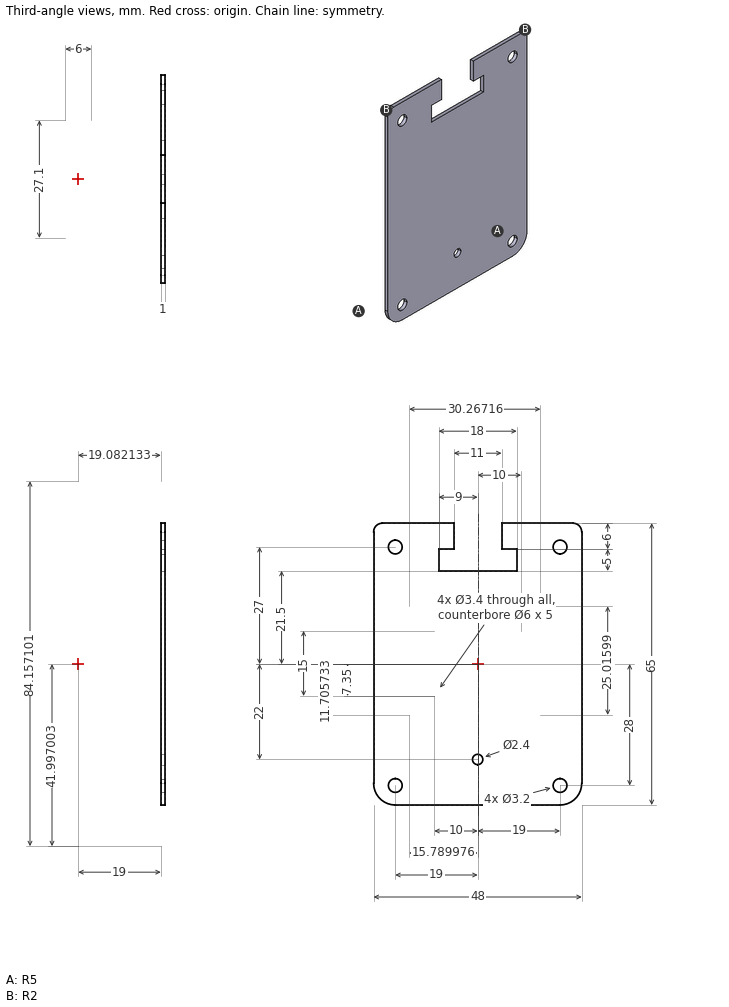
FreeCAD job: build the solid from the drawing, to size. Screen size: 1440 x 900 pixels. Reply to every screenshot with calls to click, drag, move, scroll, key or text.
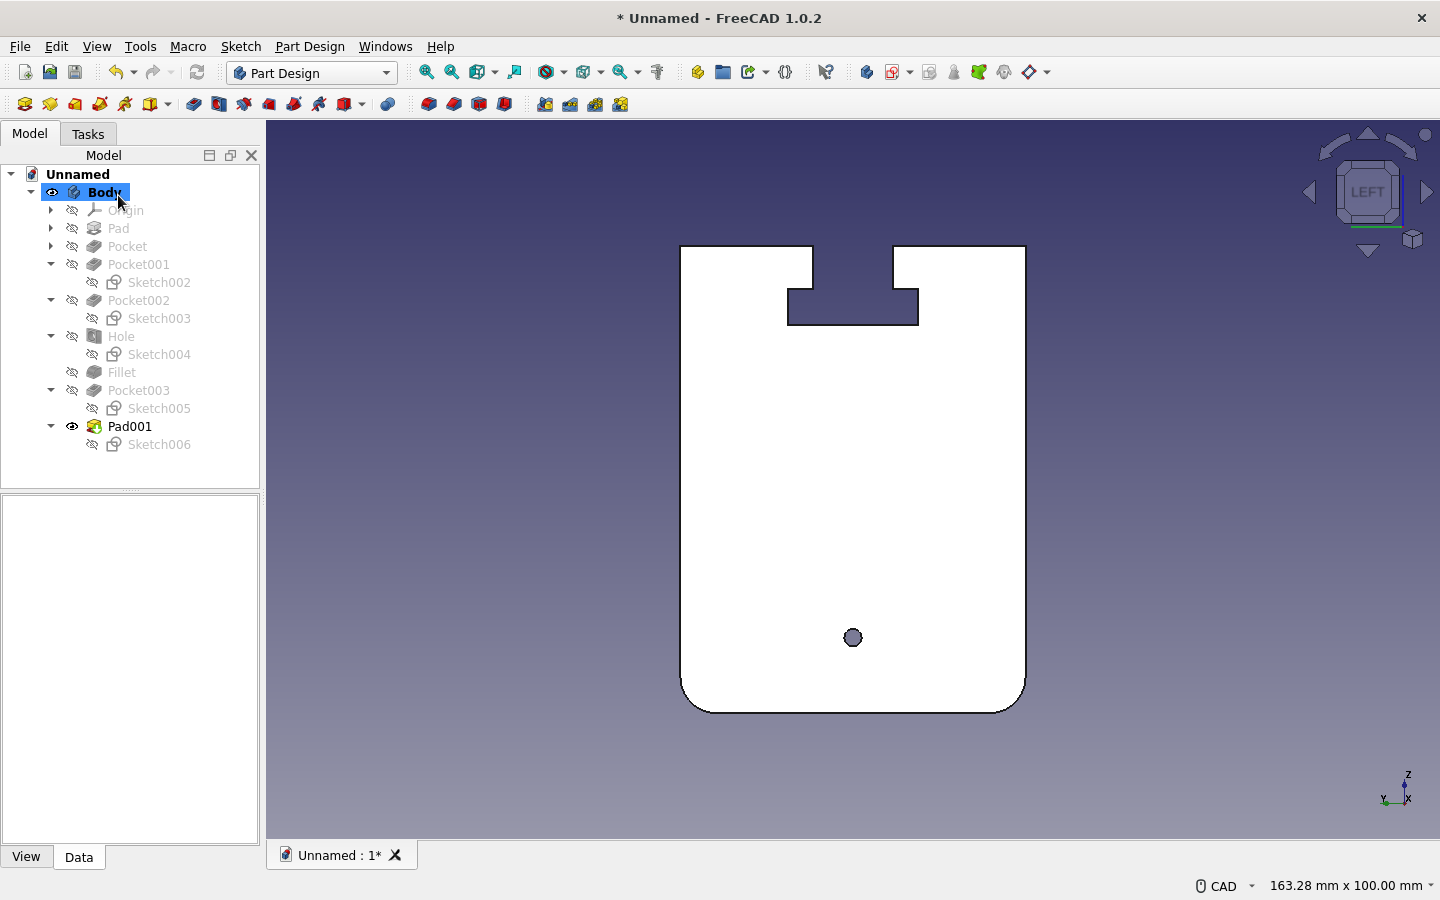
click(853, 479)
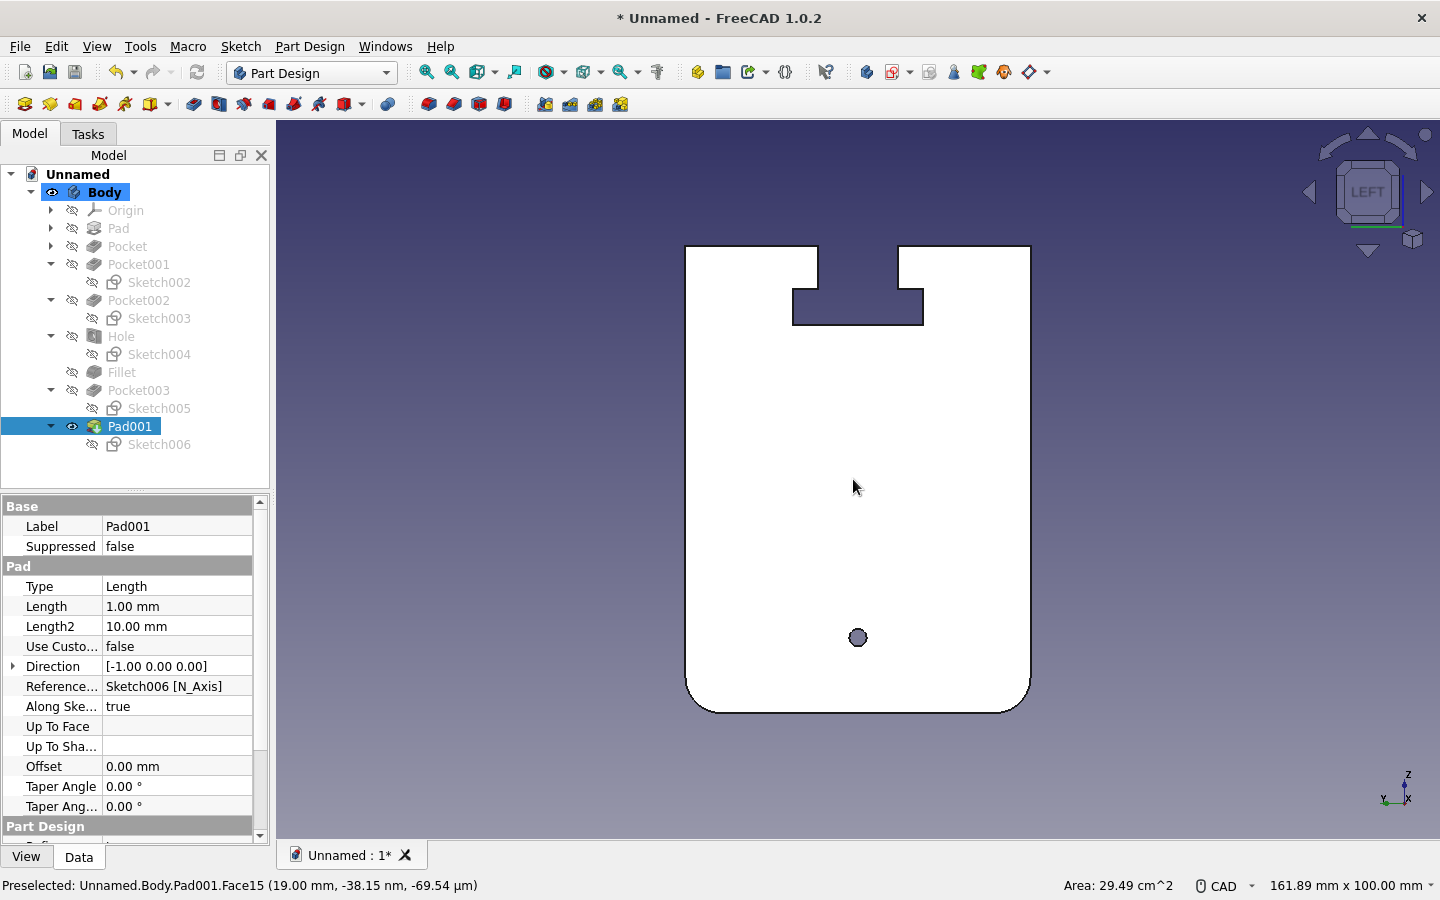
click(892, 72)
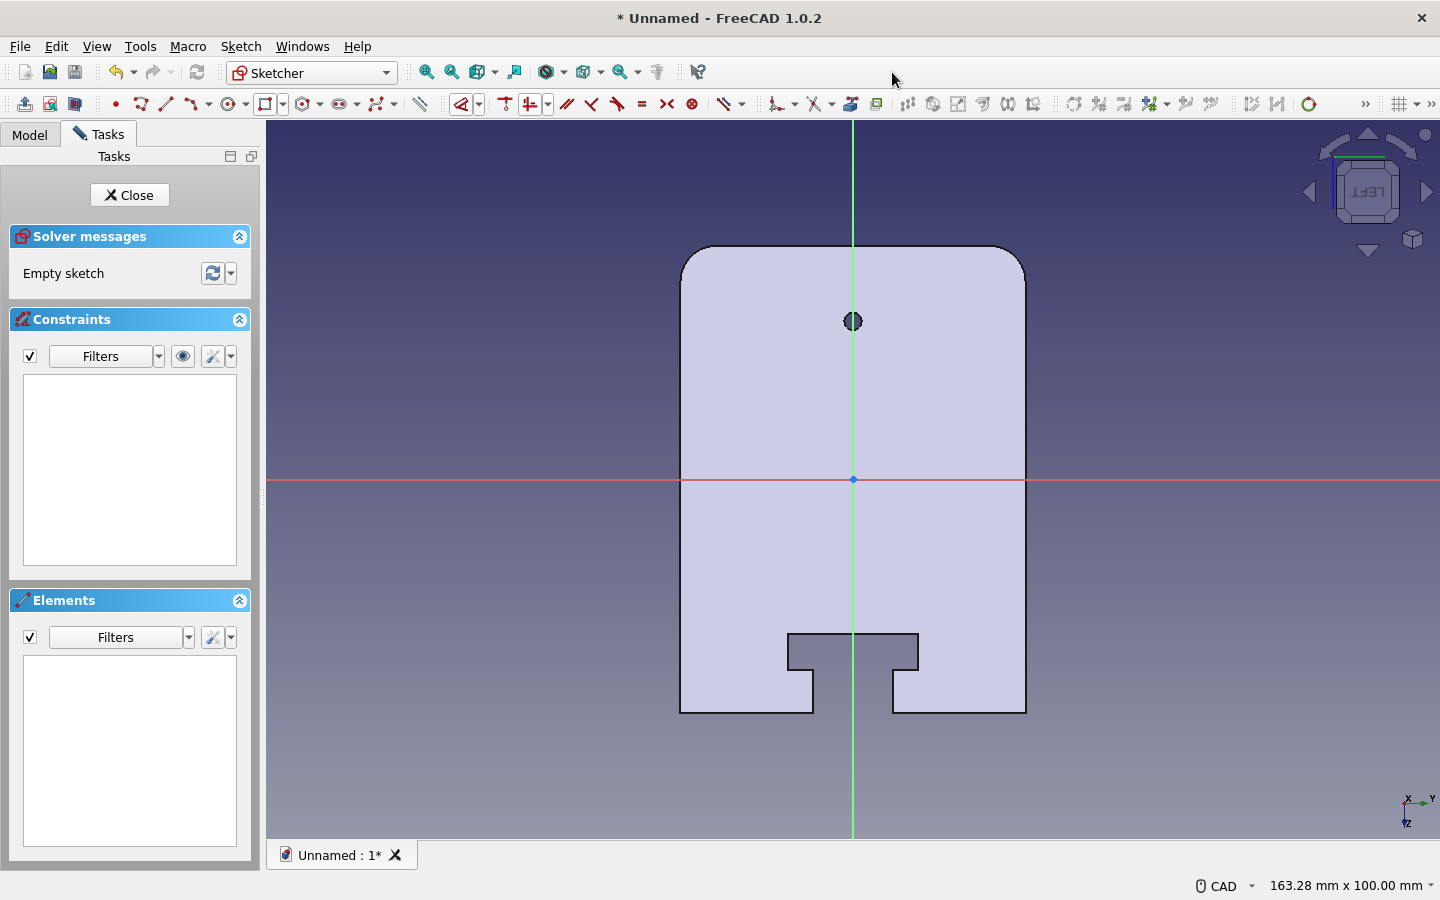
key(g)
key(c)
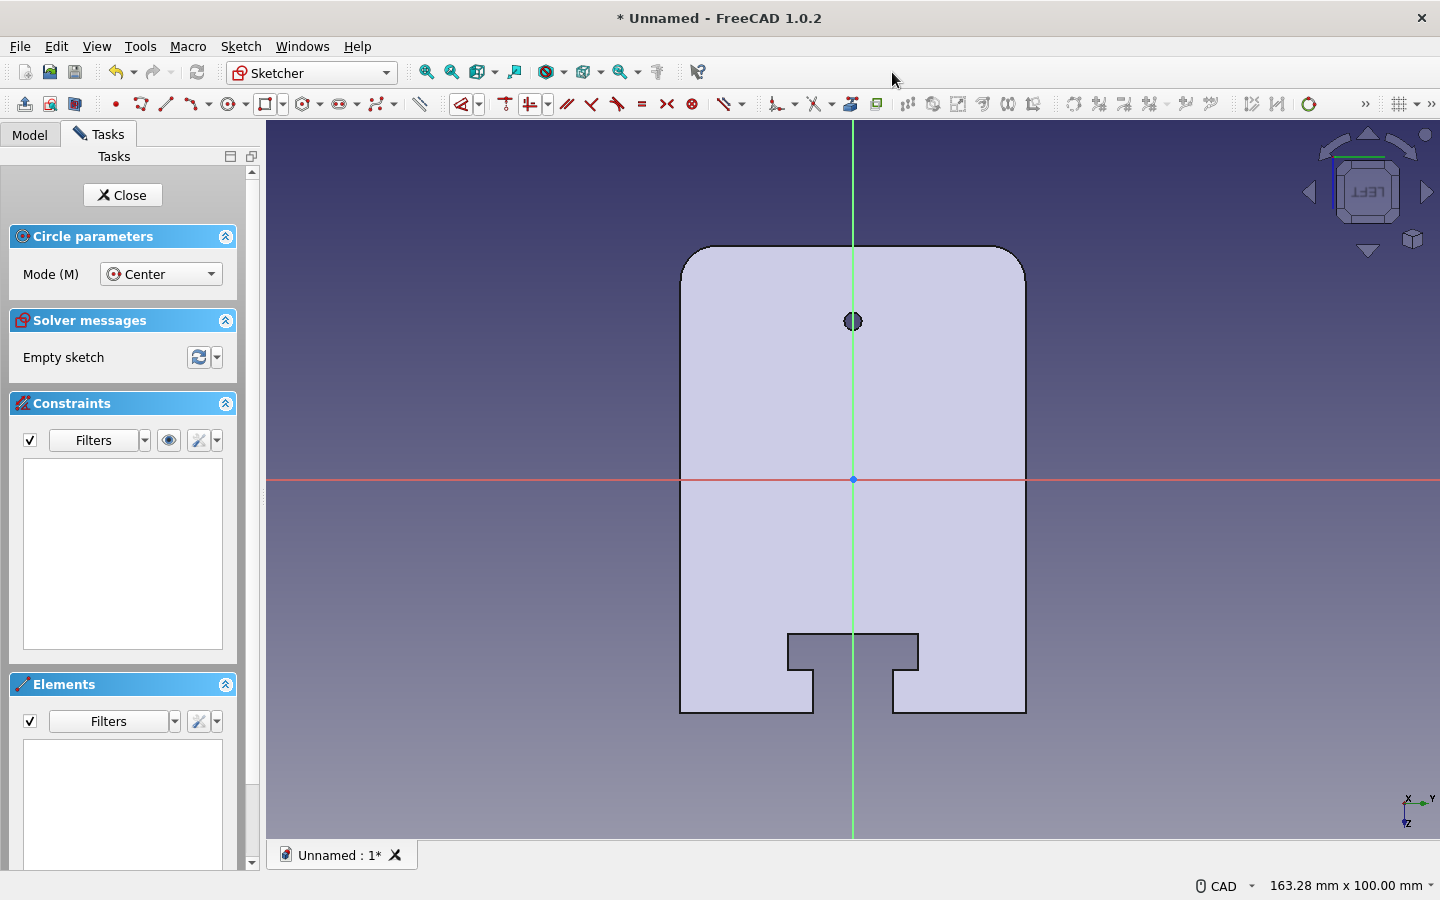
scroll(990, 278, up, 4)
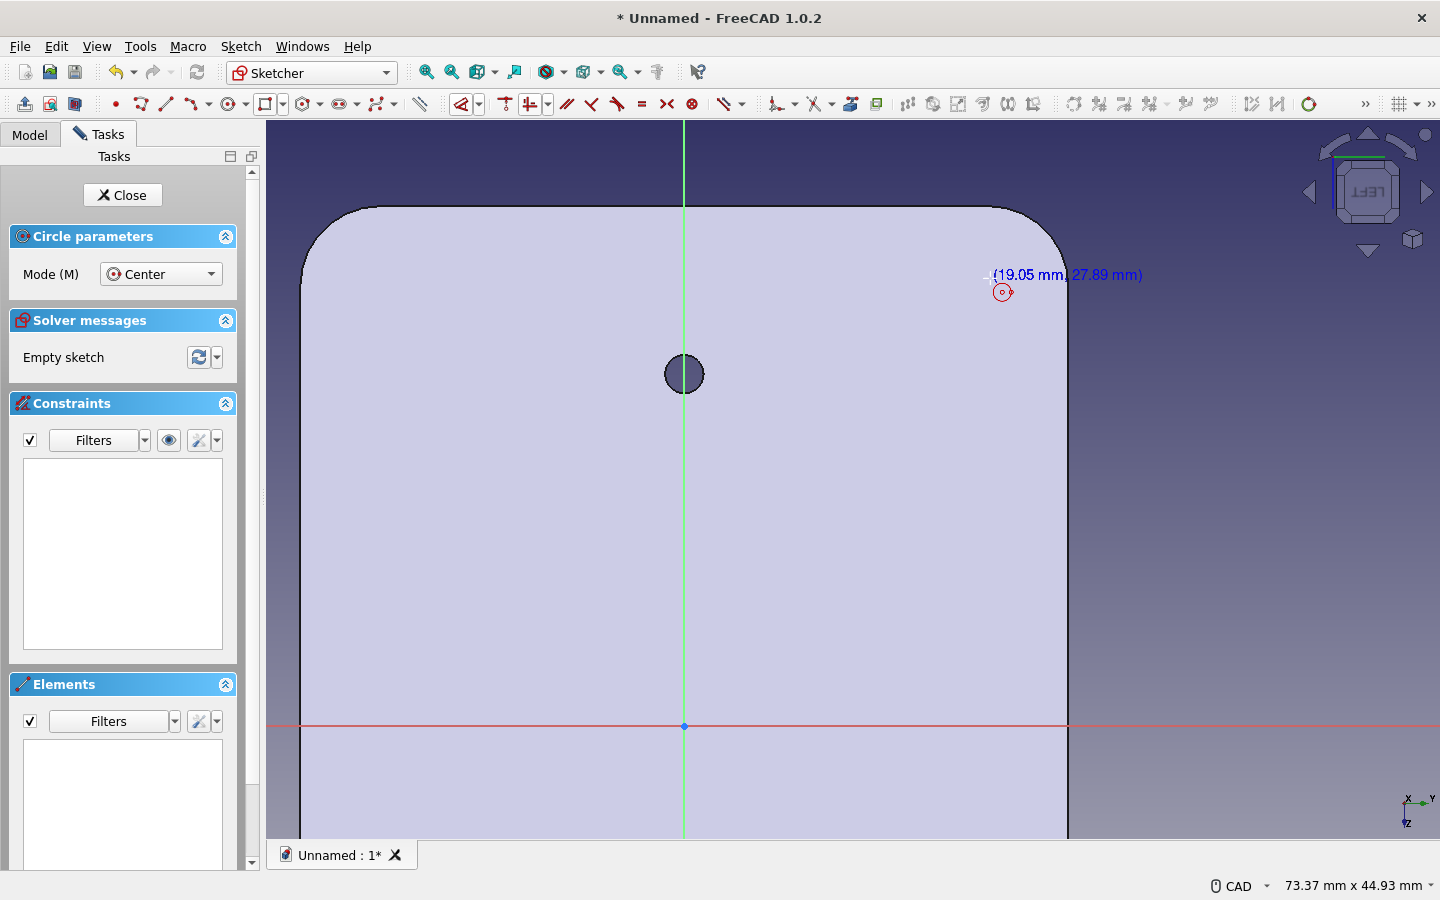
click(988, 278)
move(1006, 260)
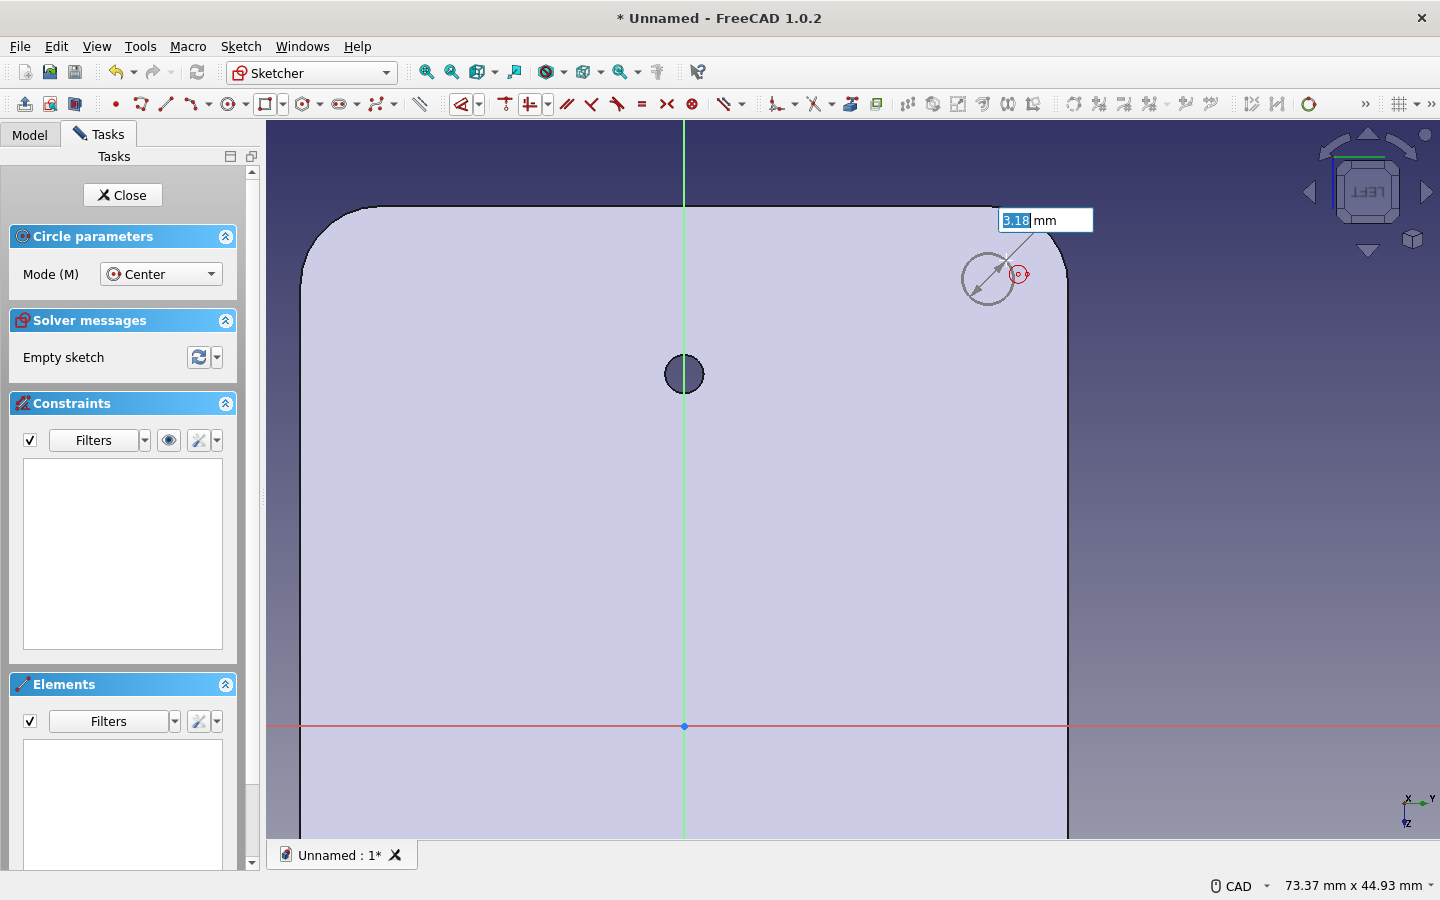
text(3.2)
key(Return)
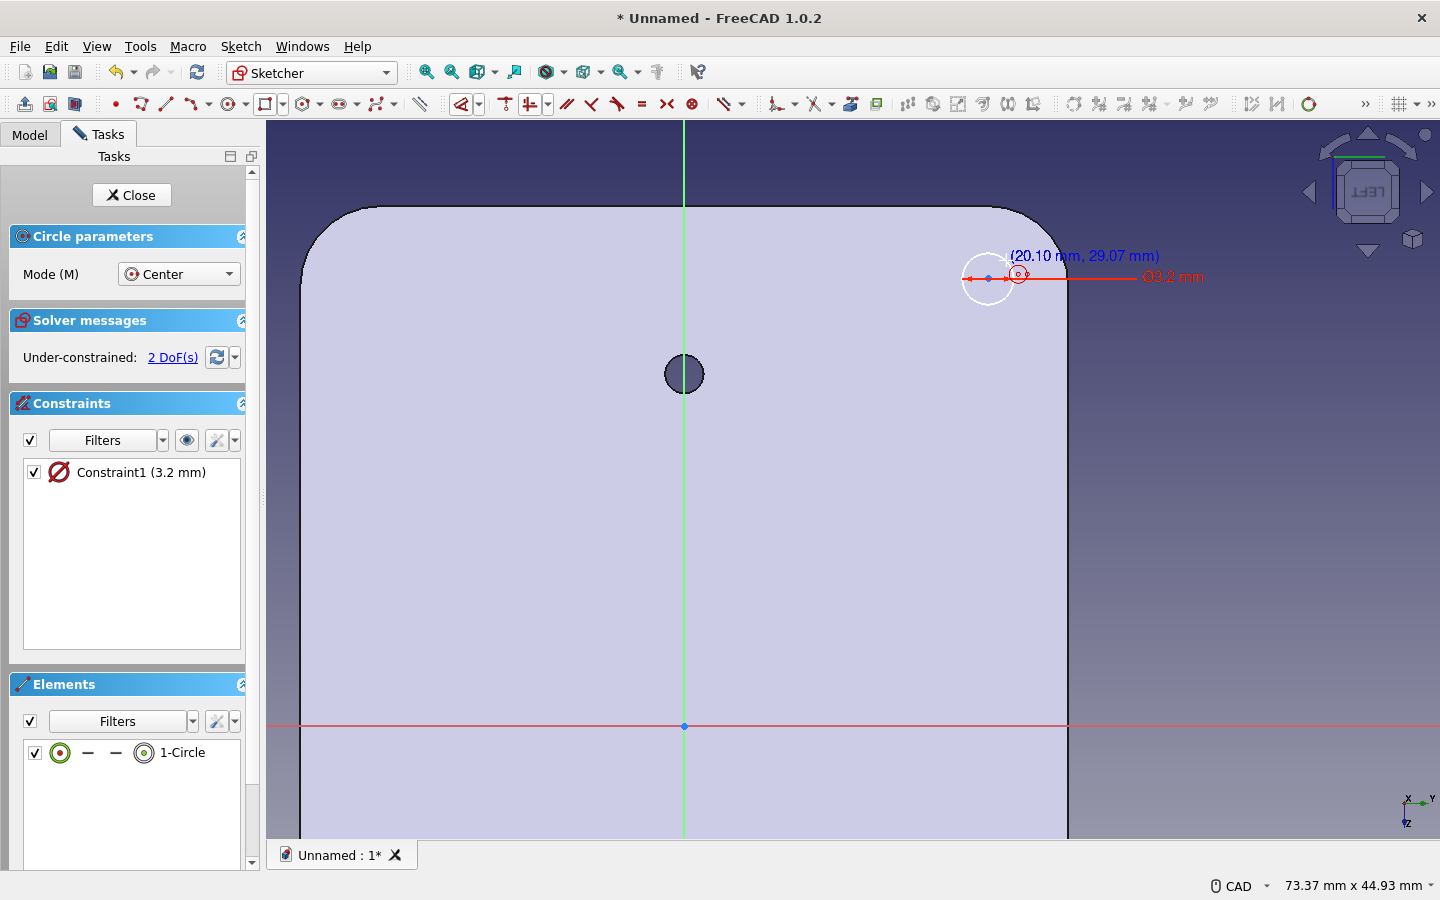
click(380, 278)
move(398, 260)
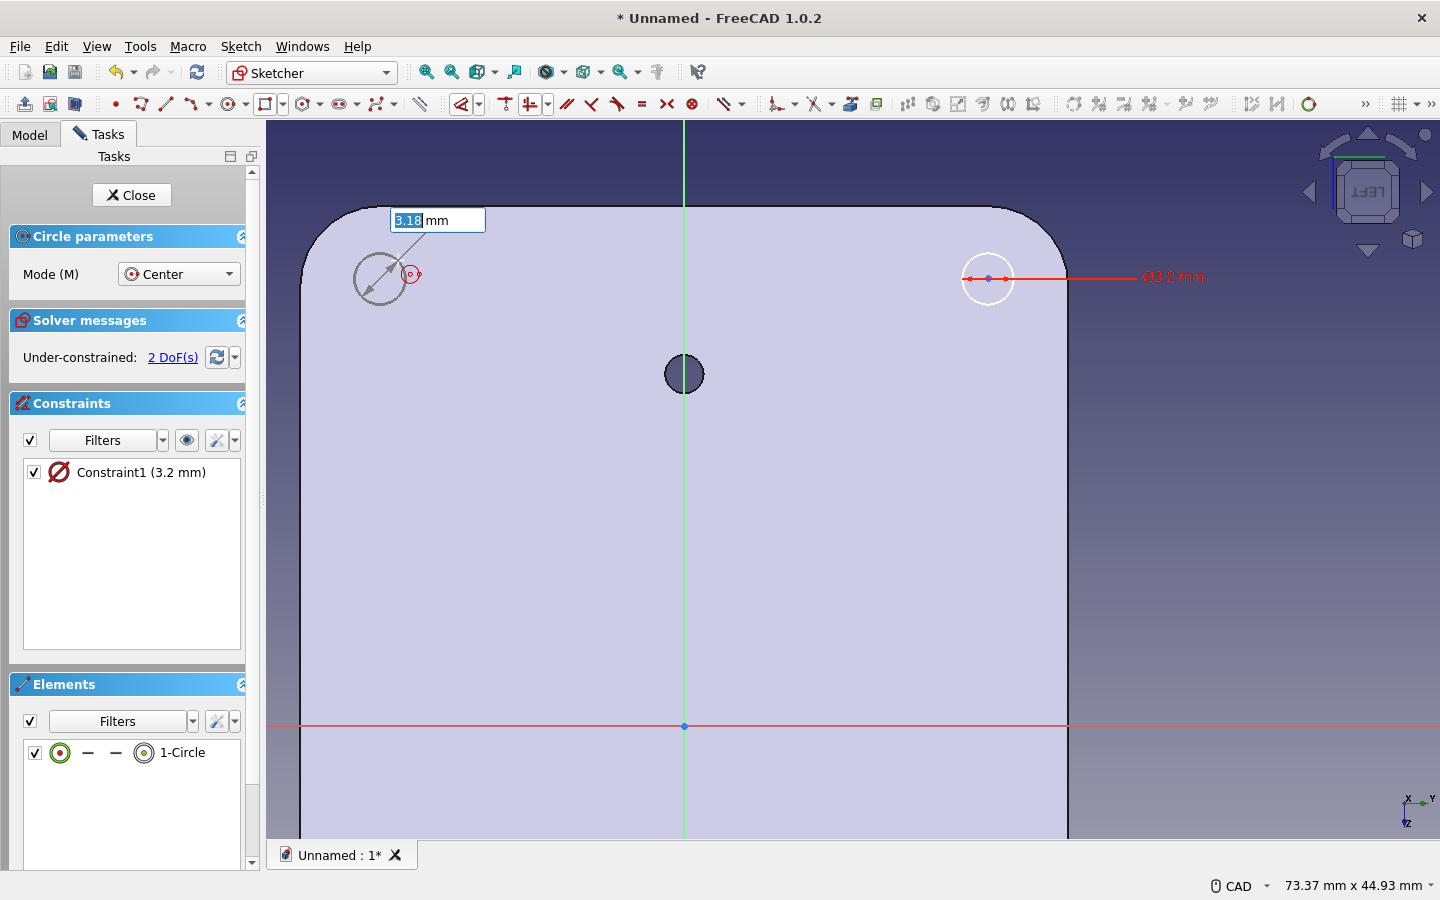
text(3.2)
key(Return)